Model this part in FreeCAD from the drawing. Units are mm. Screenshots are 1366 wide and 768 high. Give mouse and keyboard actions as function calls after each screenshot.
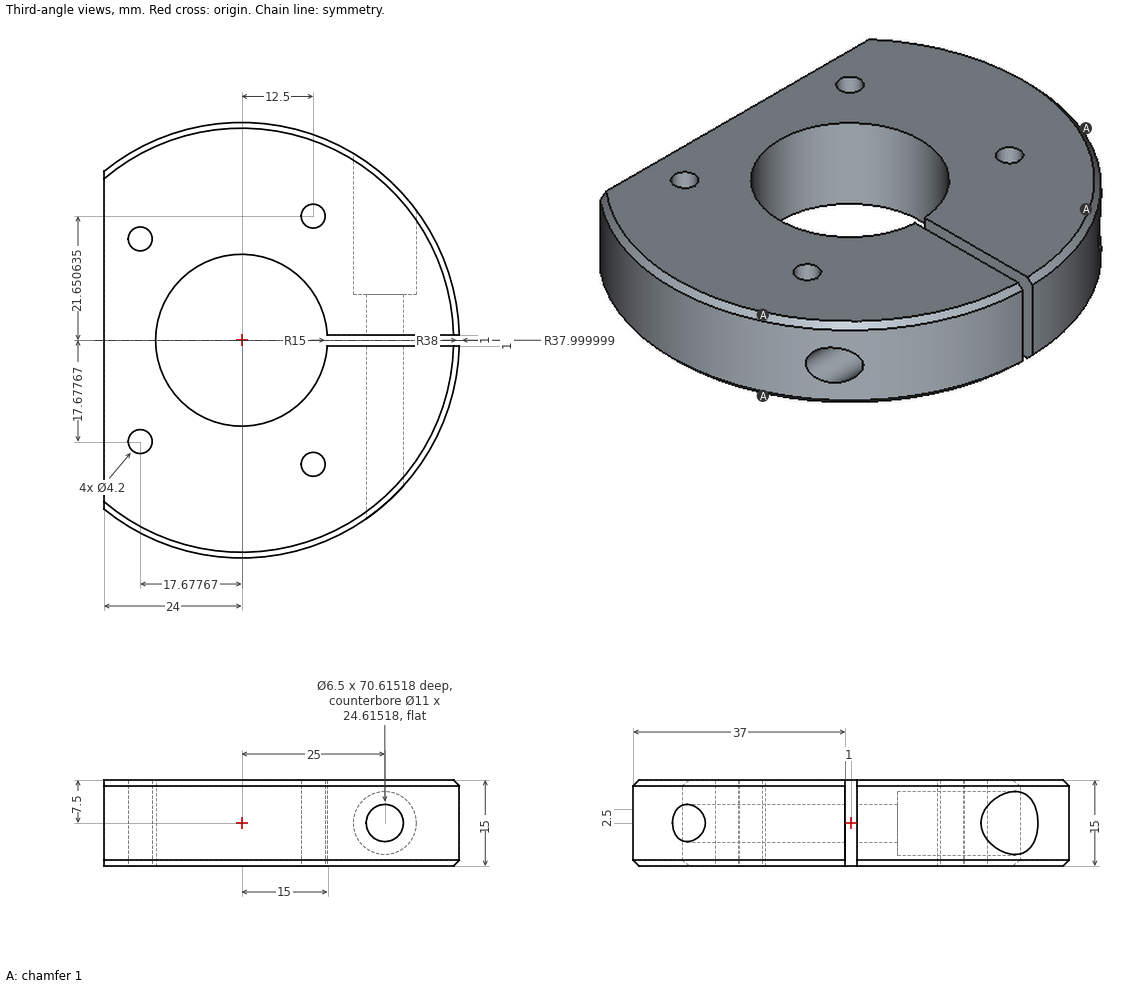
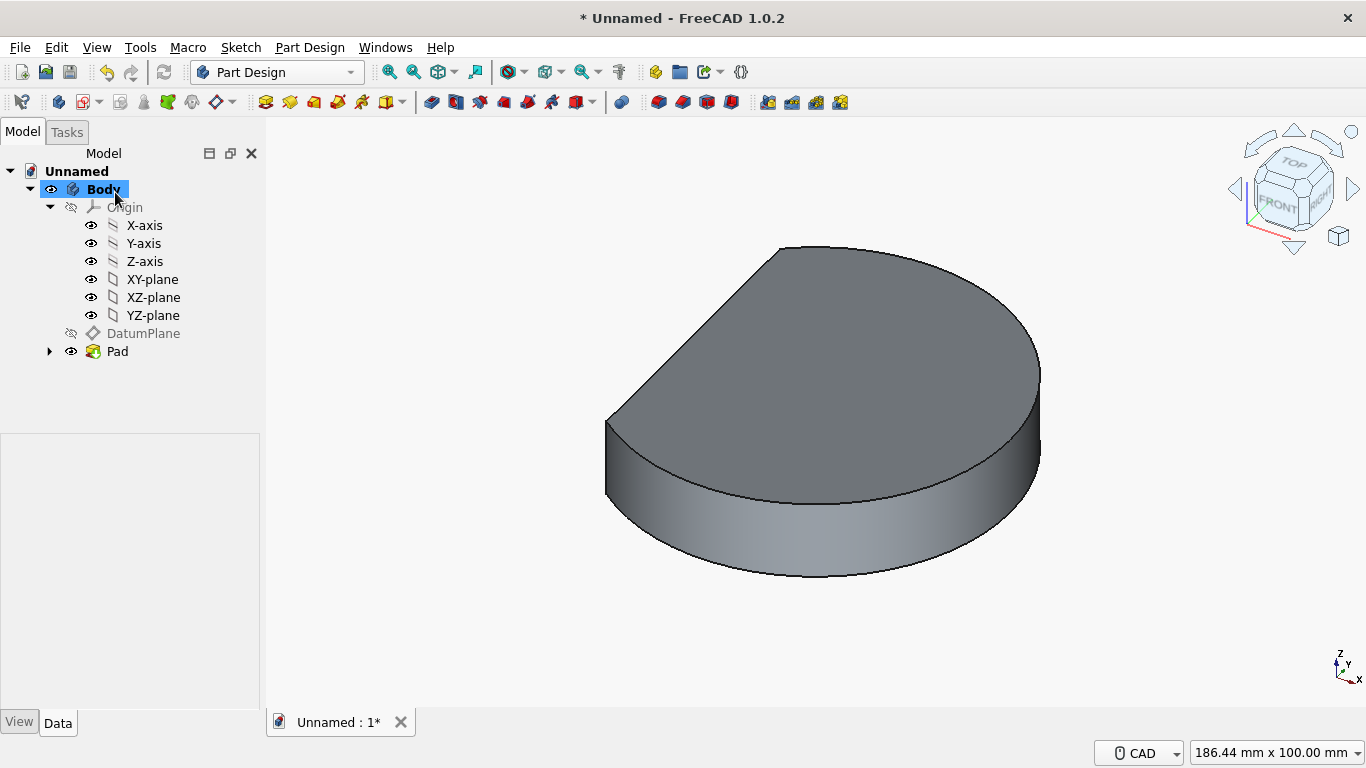
click(852, 387)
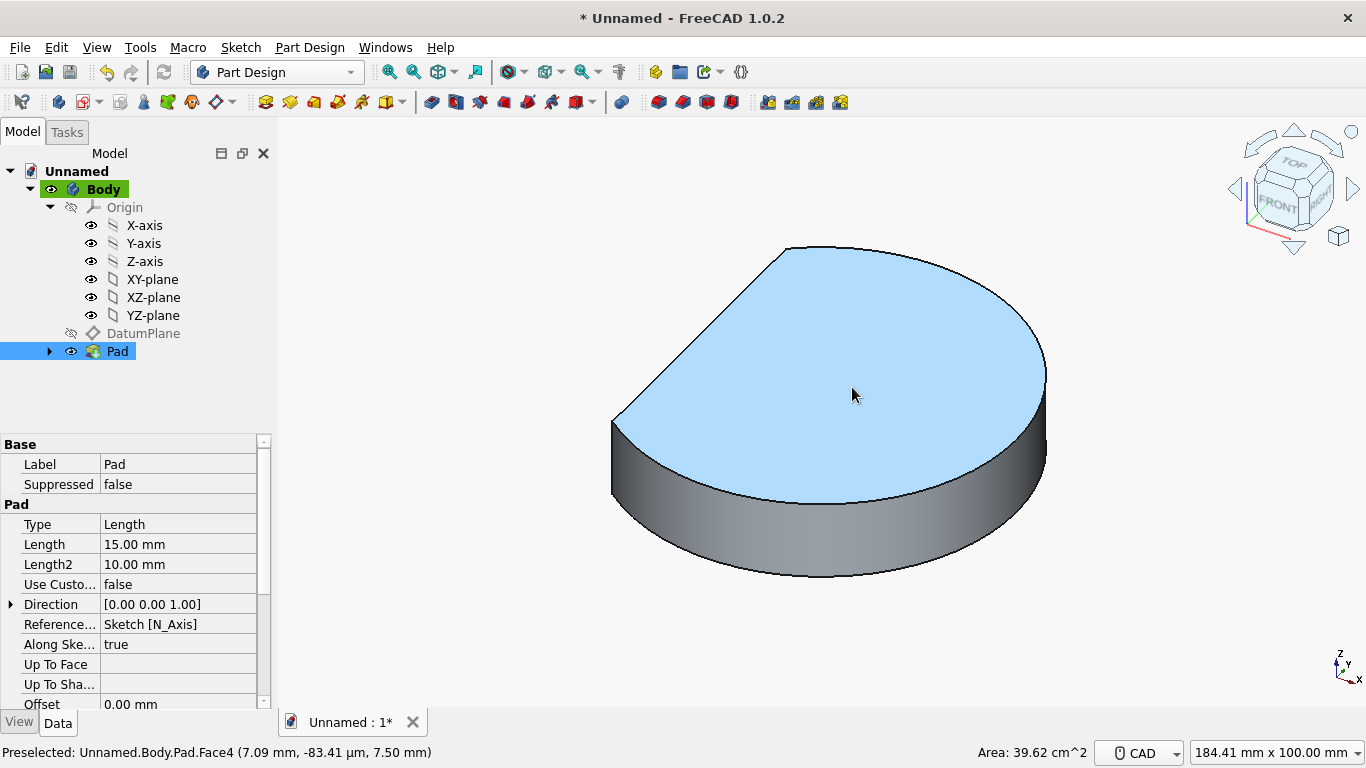
click(84, 102)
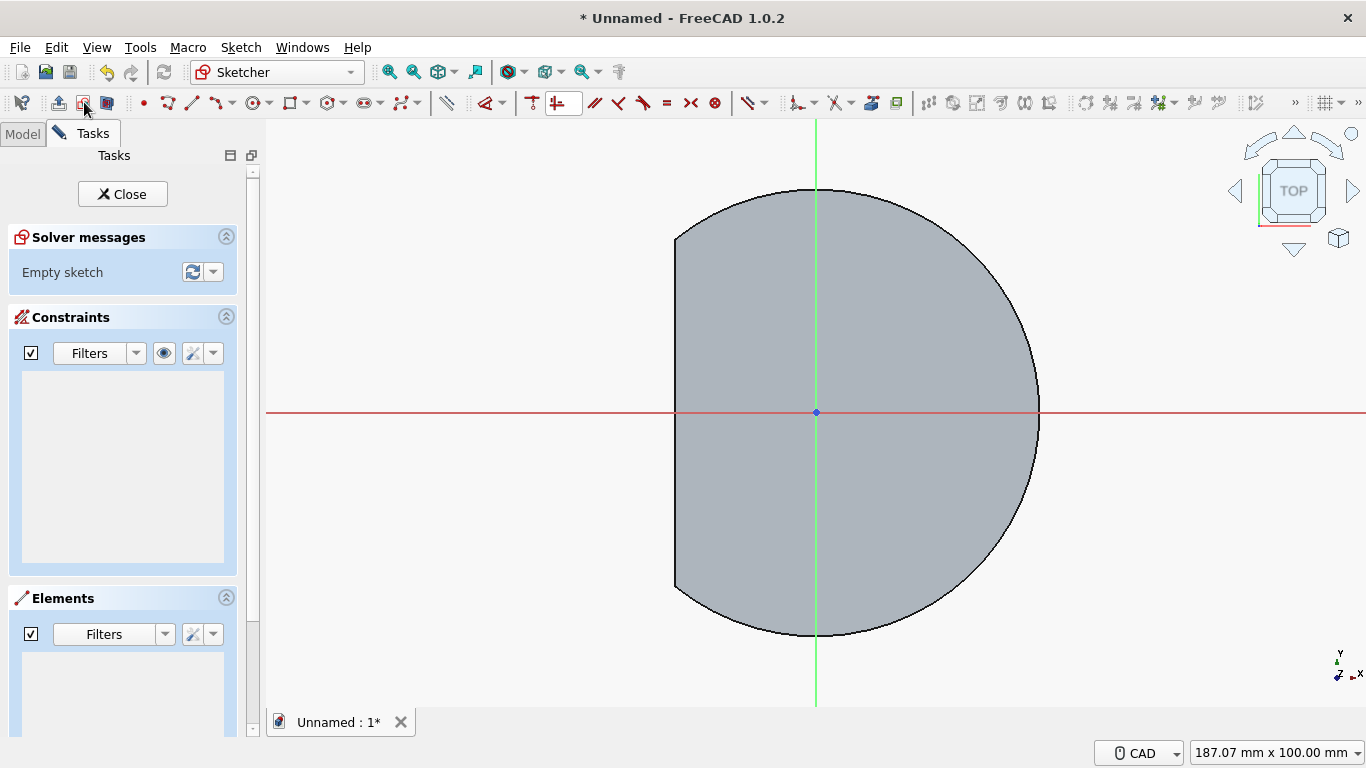
scroll(1033, 413, up, 5)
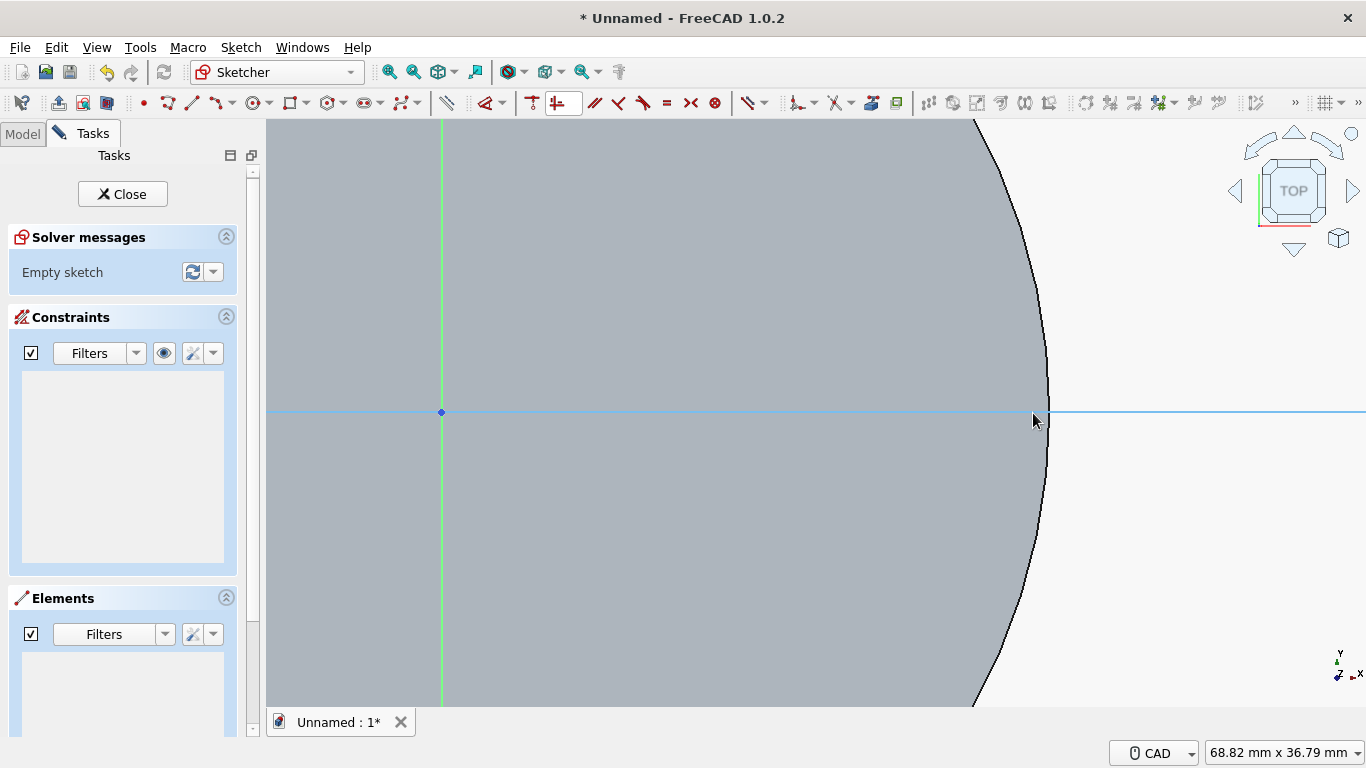
click(192, 104)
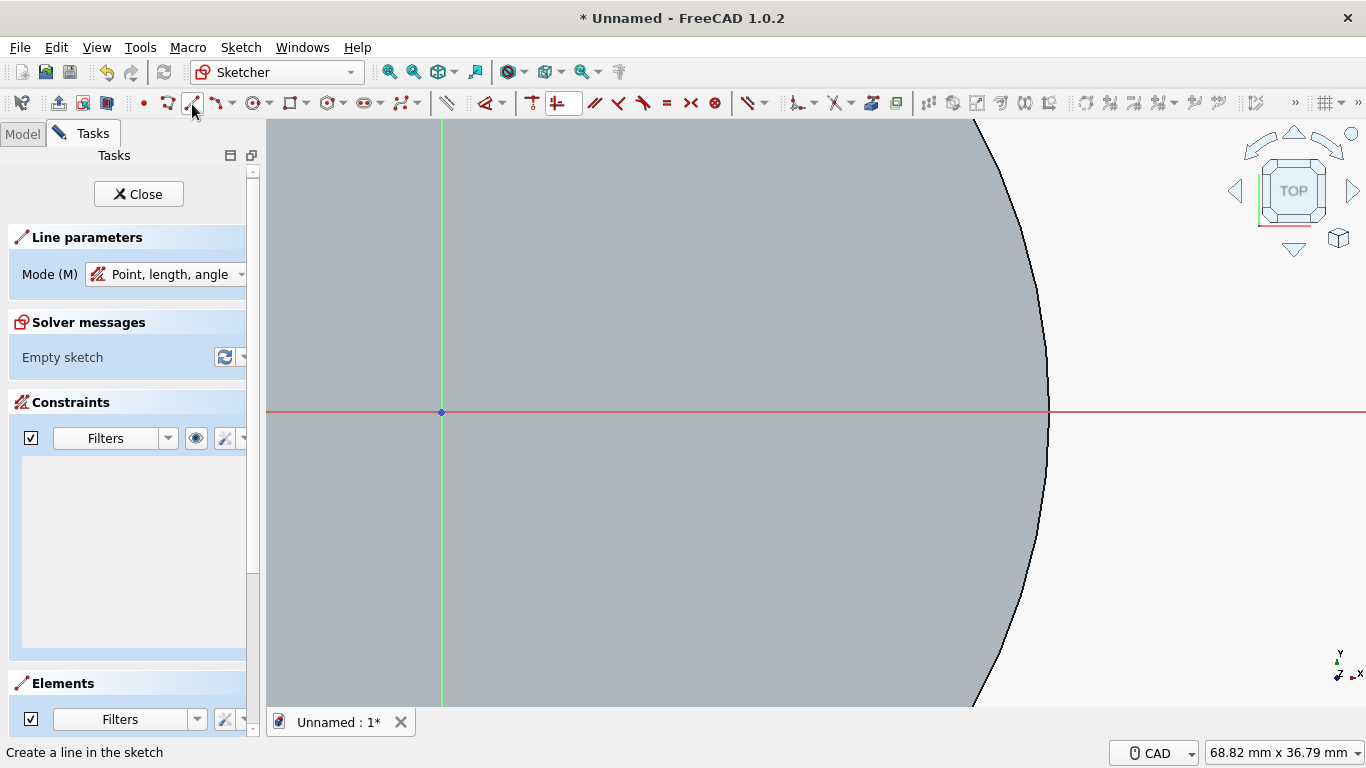
click(1049, 396)
click(681, 396)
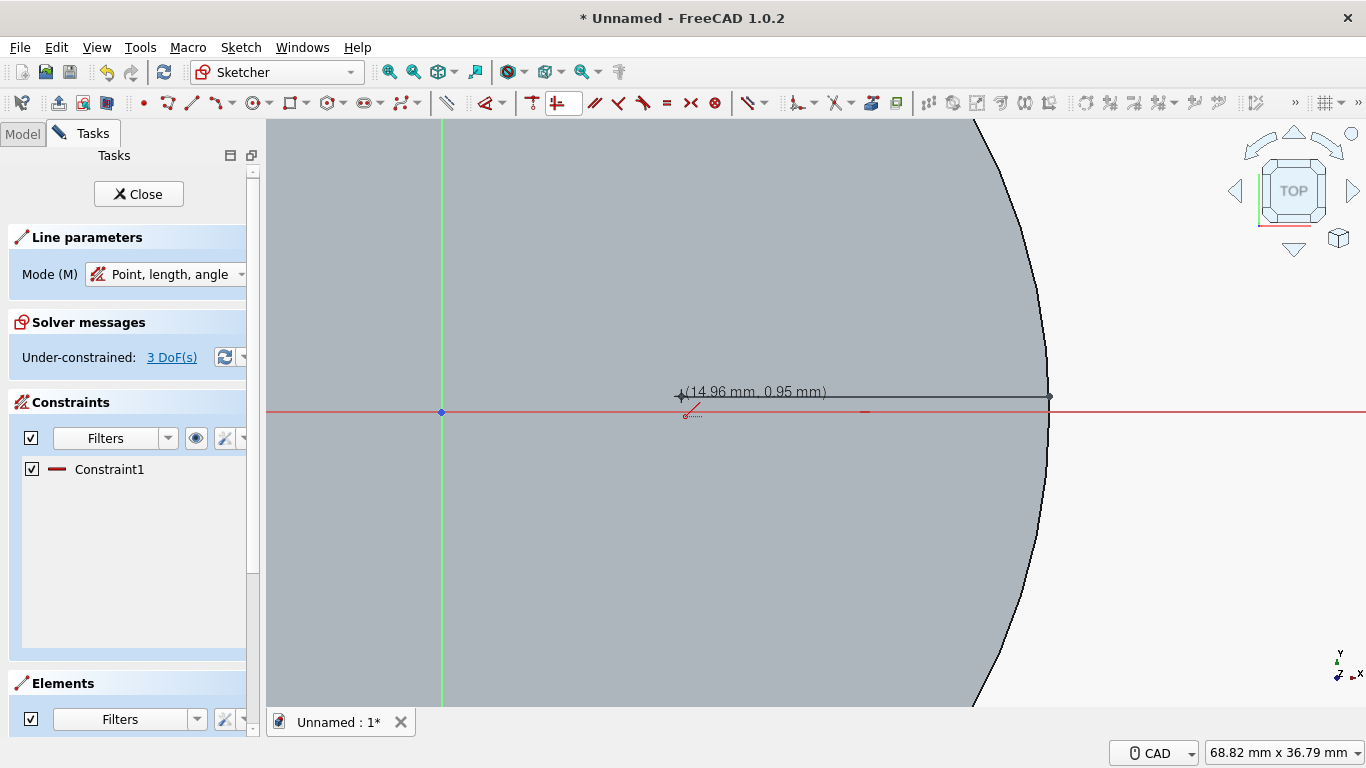
click(681, 428)
click(1049, 428)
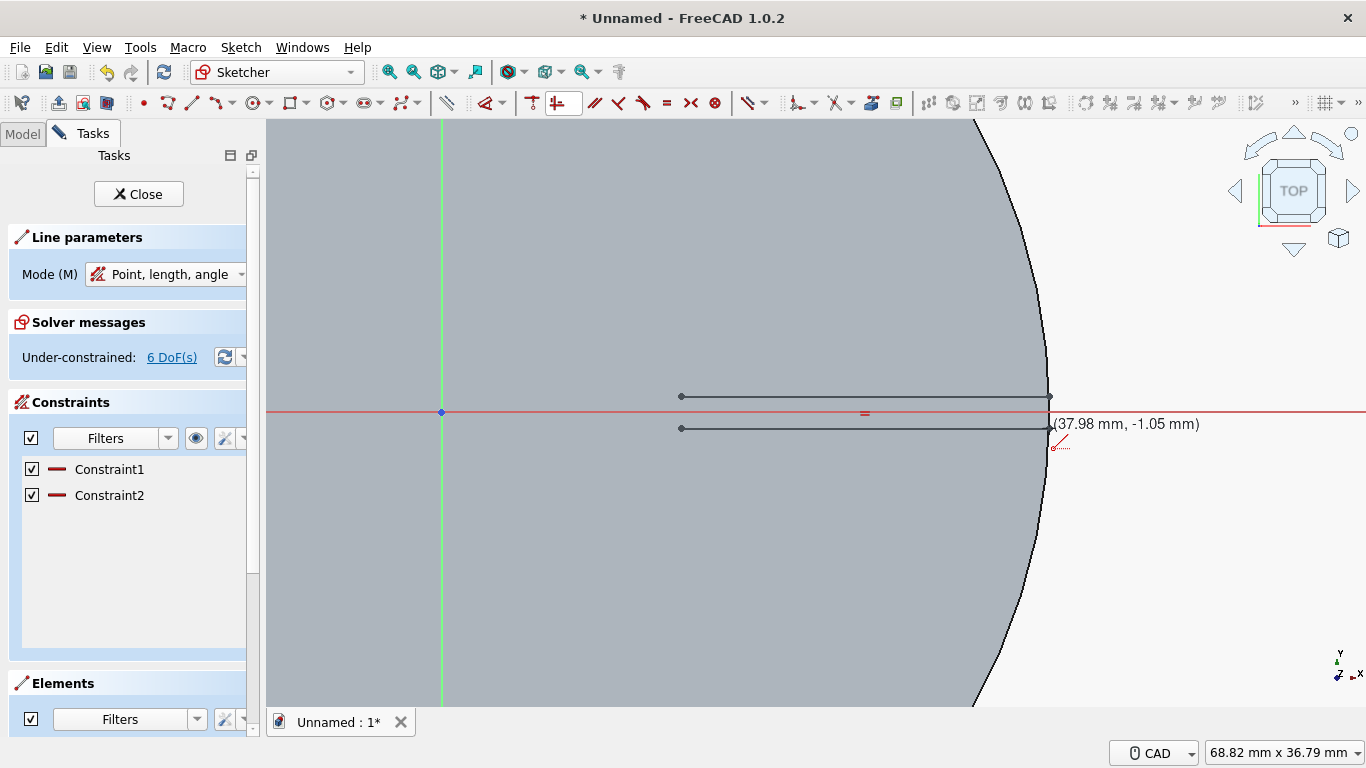
click(216, 104)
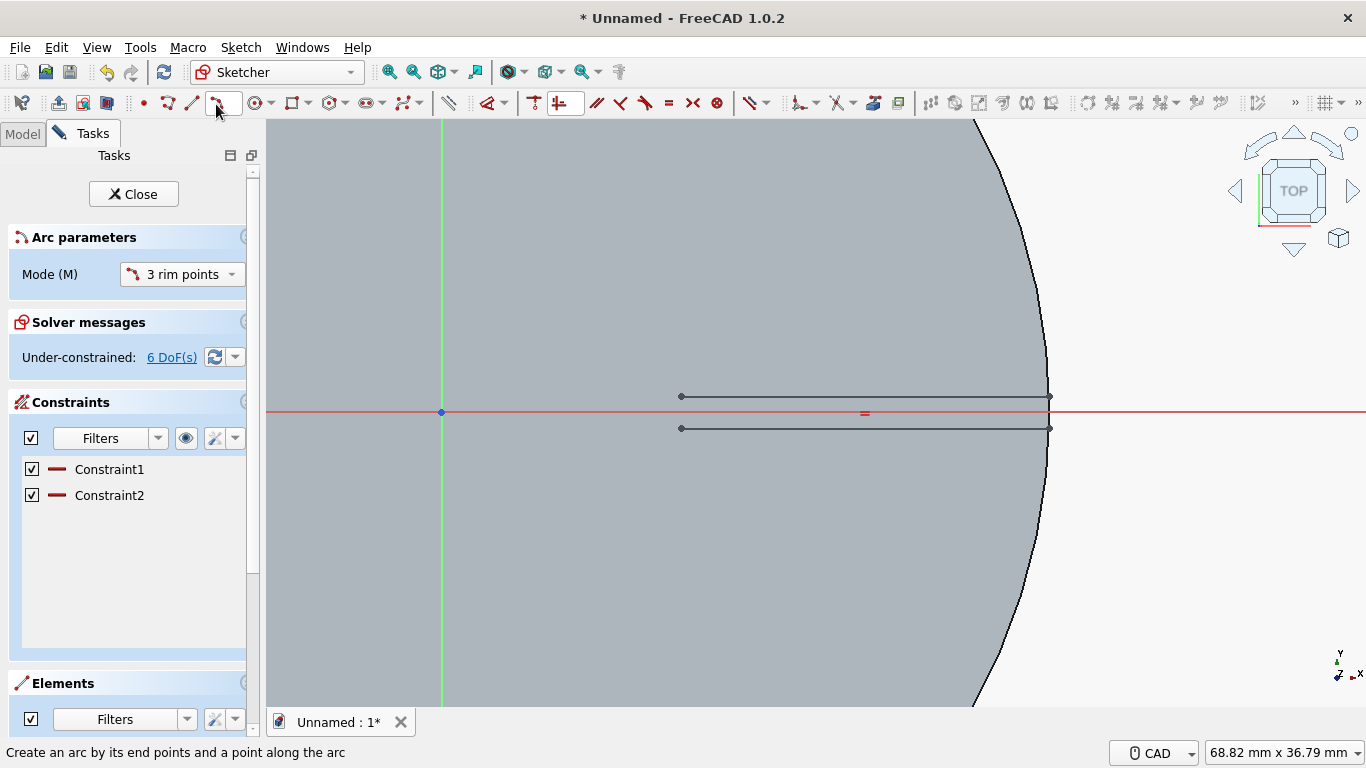
click(681, 397)
click(681, 429)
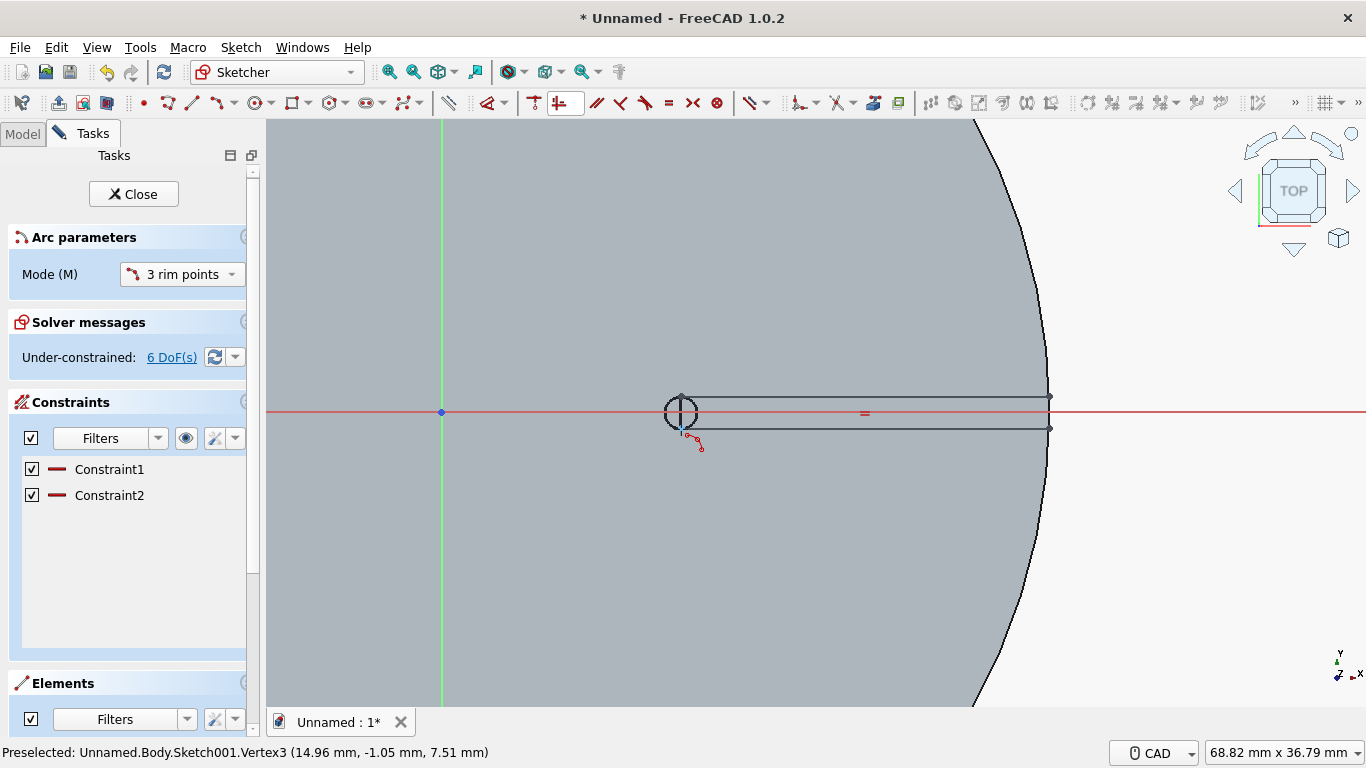
scroll(682, 415, up, 18)